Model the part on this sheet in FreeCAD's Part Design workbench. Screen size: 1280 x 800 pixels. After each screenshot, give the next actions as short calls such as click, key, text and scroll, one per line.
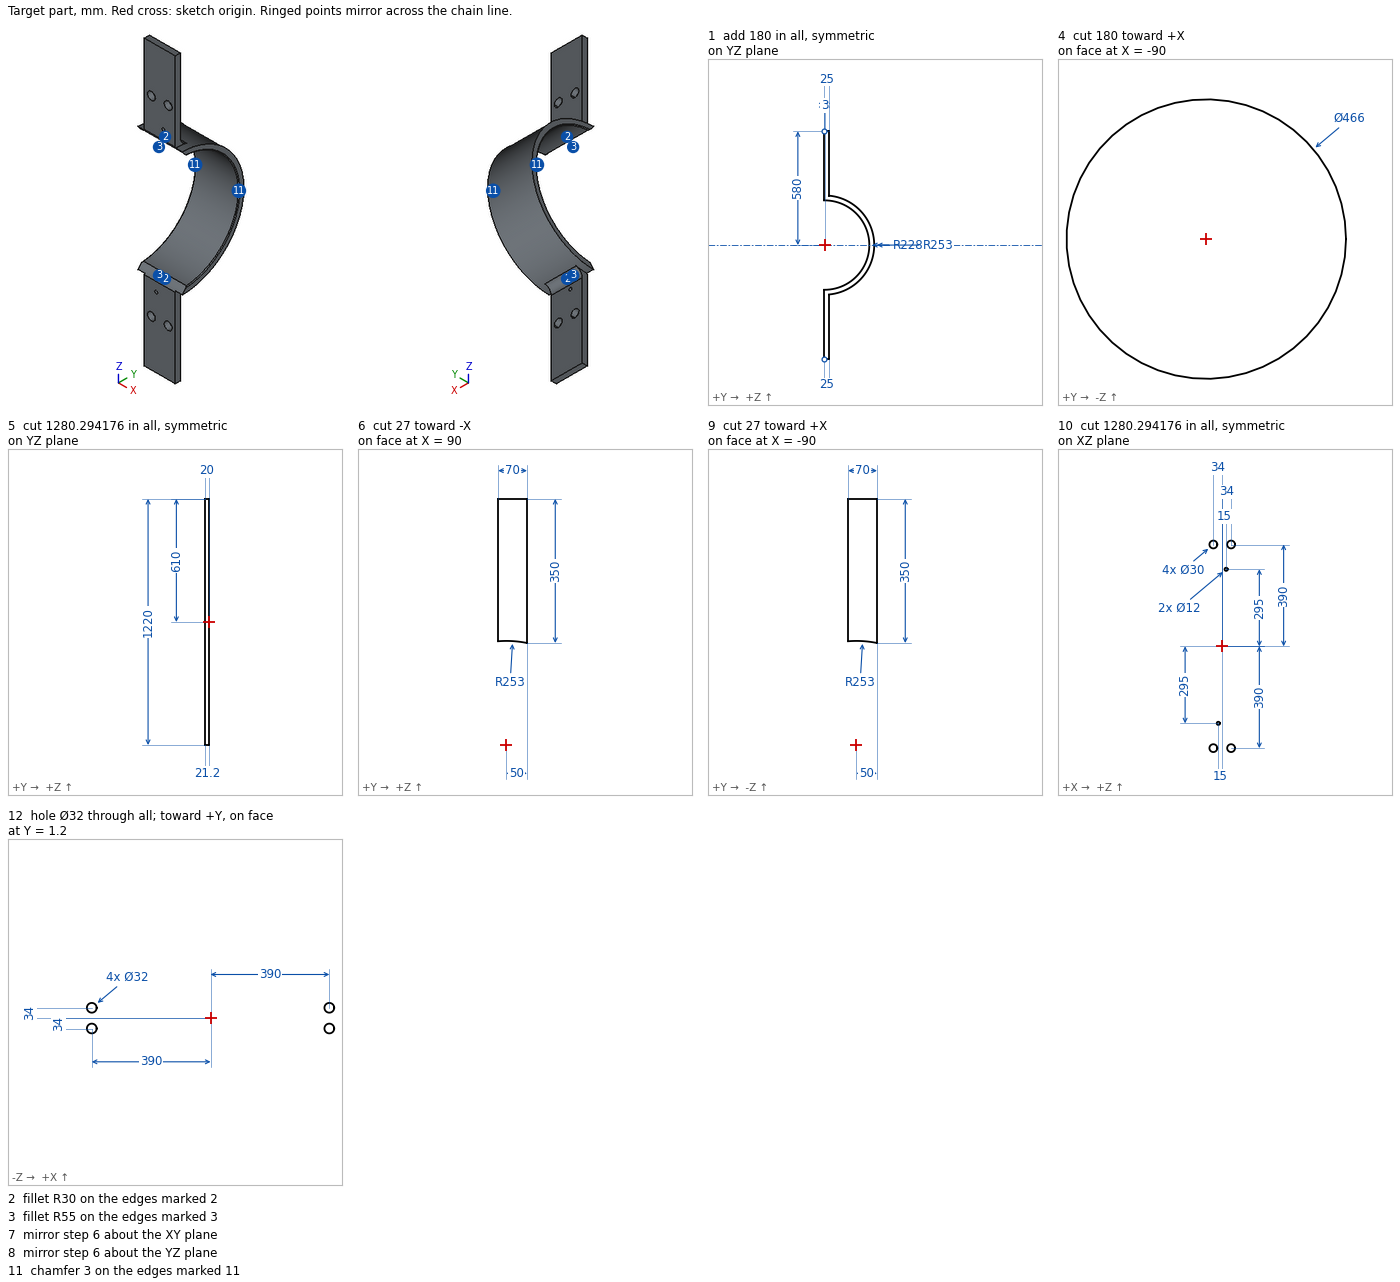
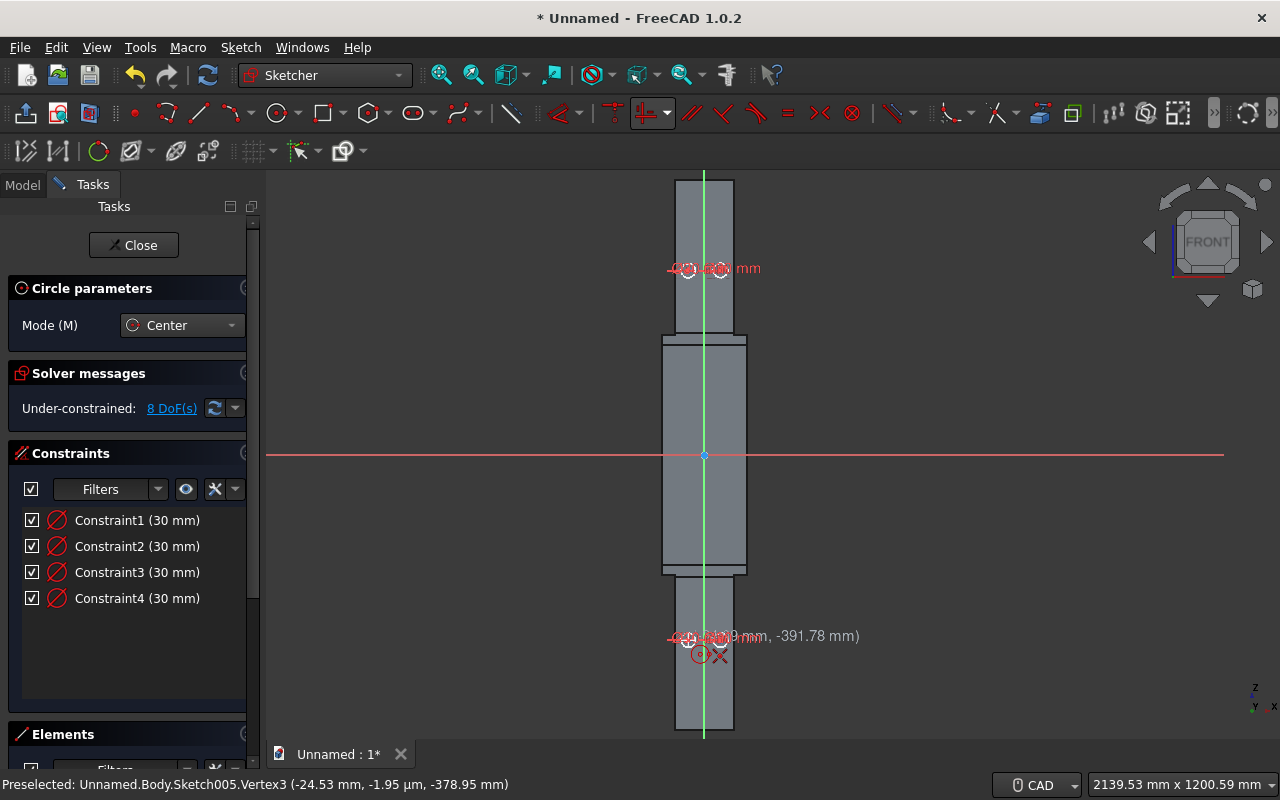
scroll(712, 315, up, 11)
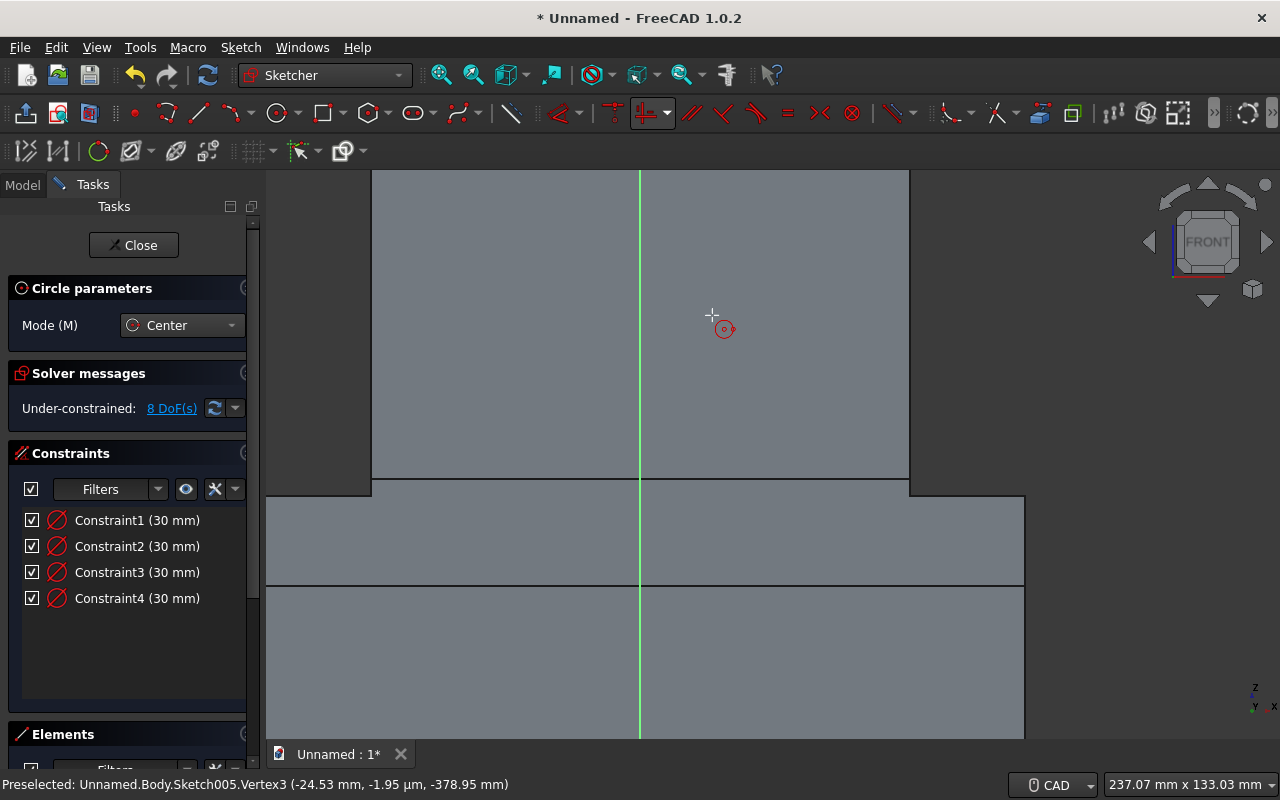
scroll(712, 314, down, 11)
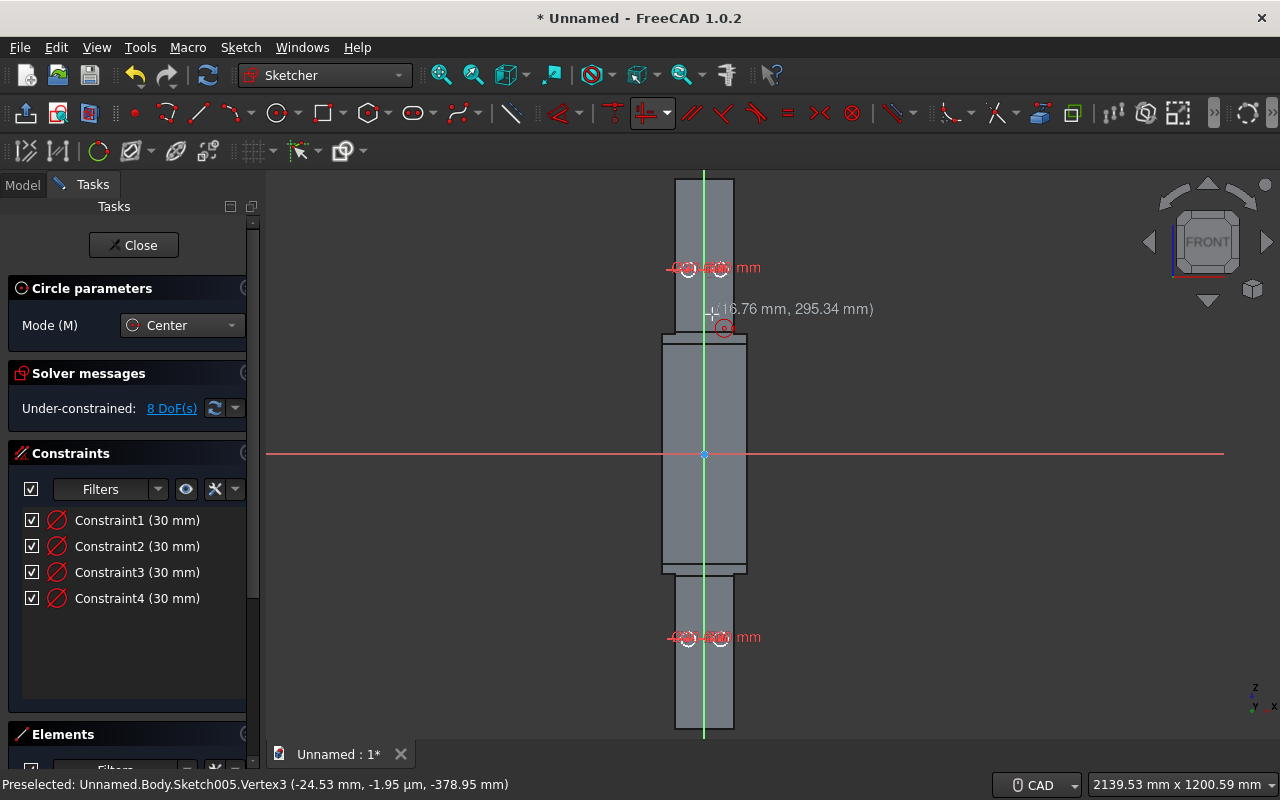
scroll(712, 314, up, 5)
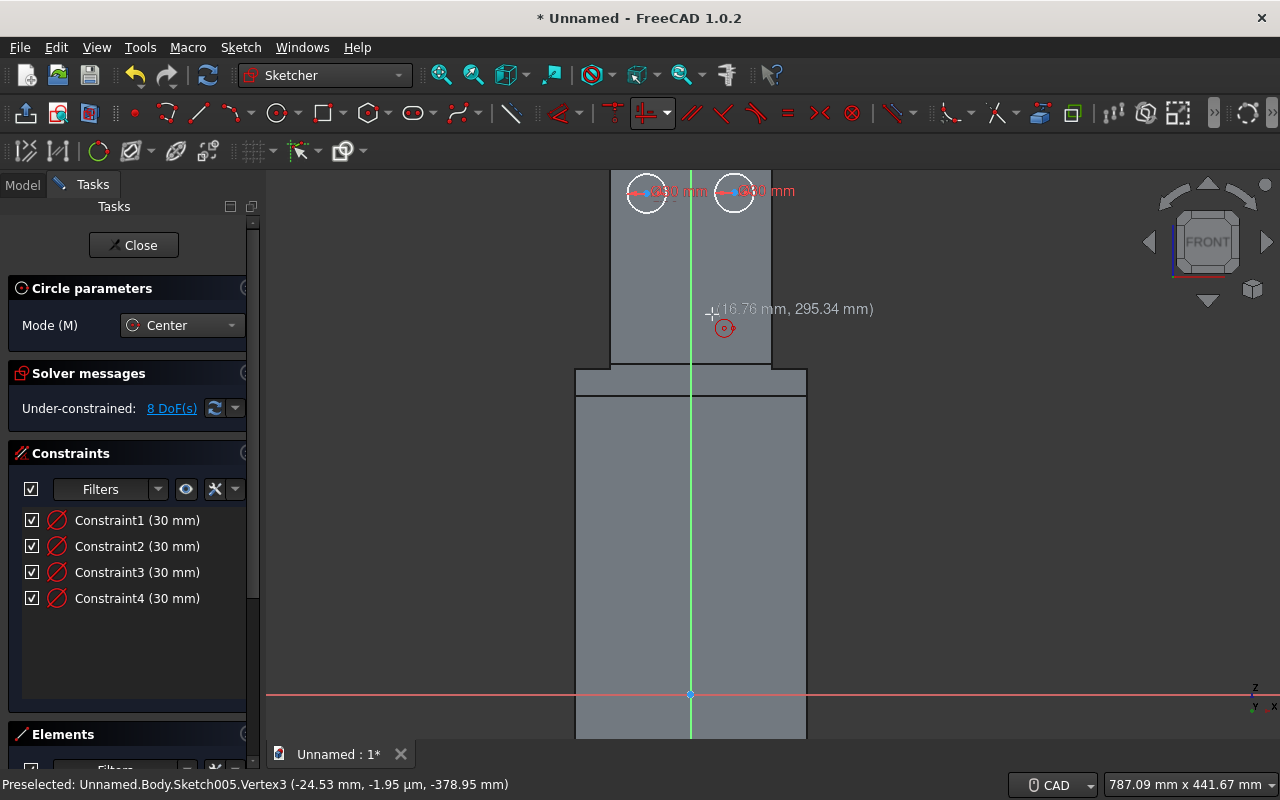
click(710, 315)
move(716, 309)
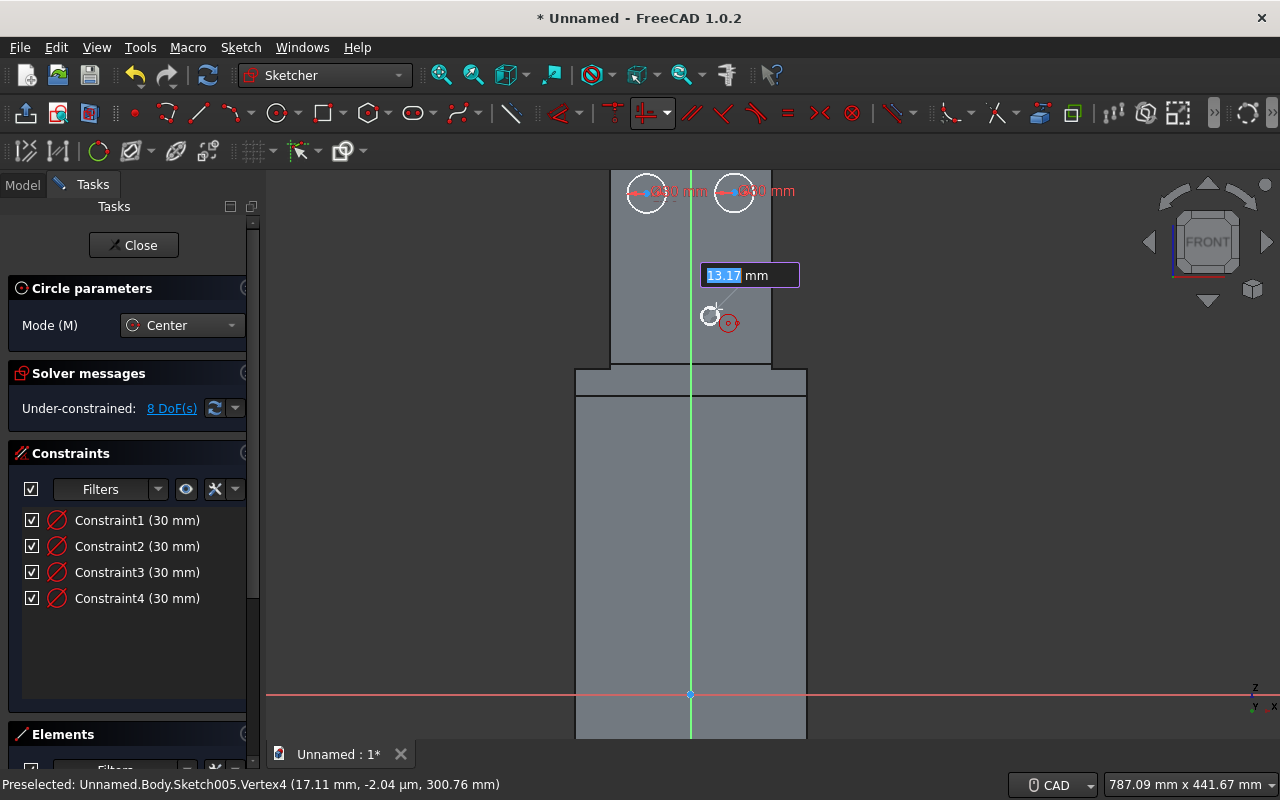
text(12)
key(Return)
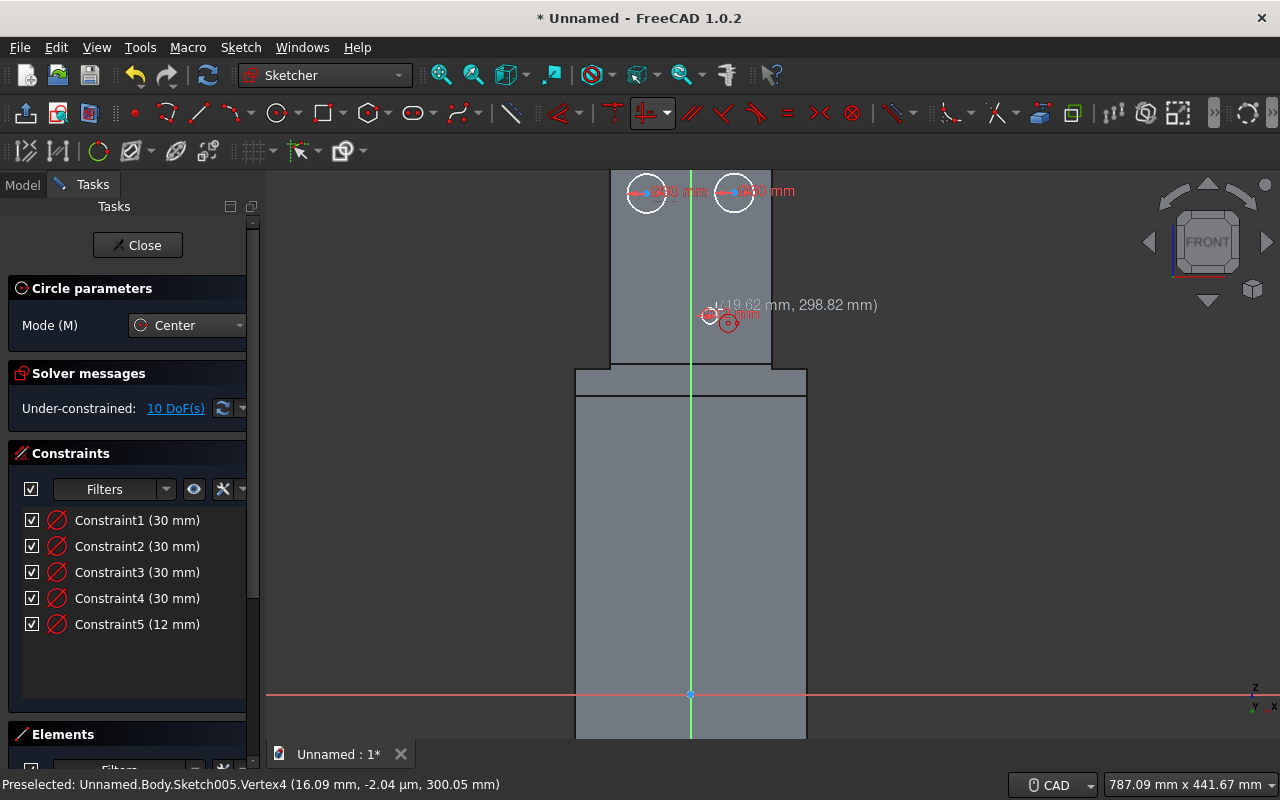
scroll(713, 315, down, 5)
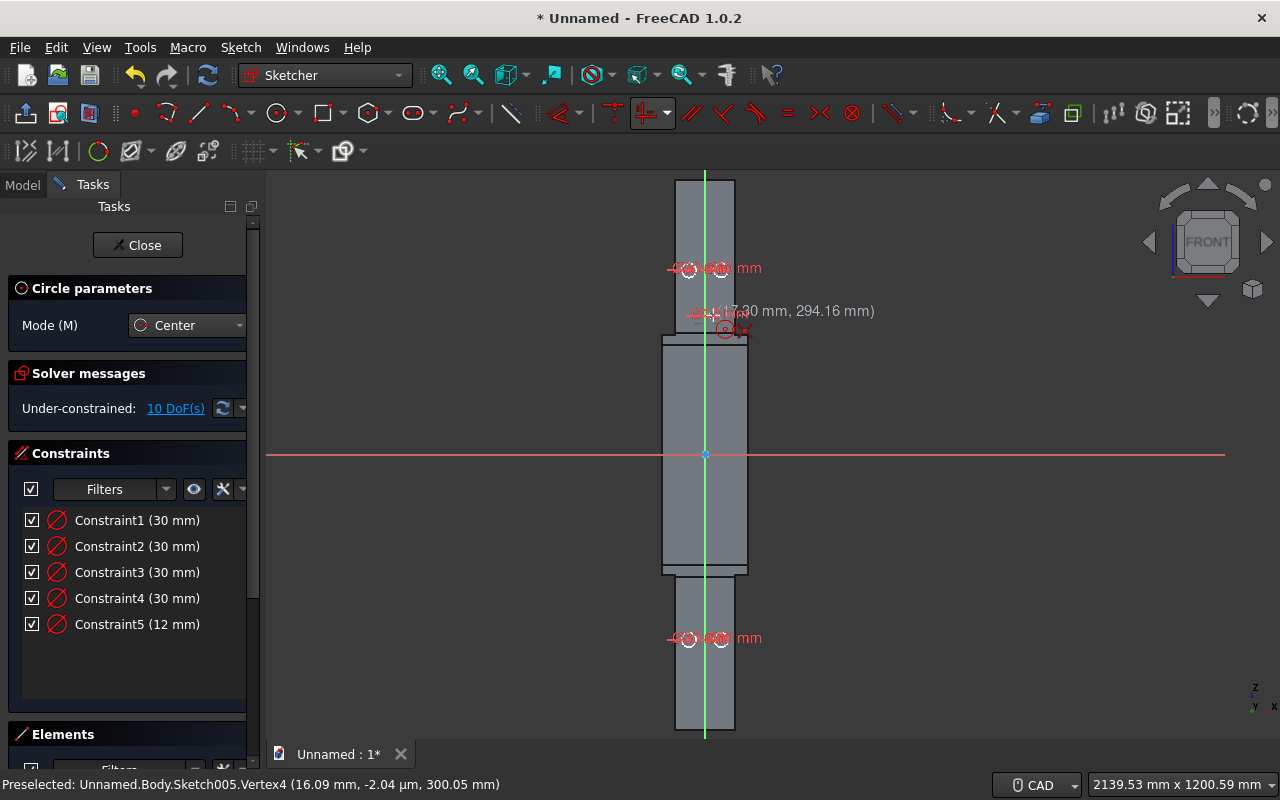
scroll(698, 595, up, 11)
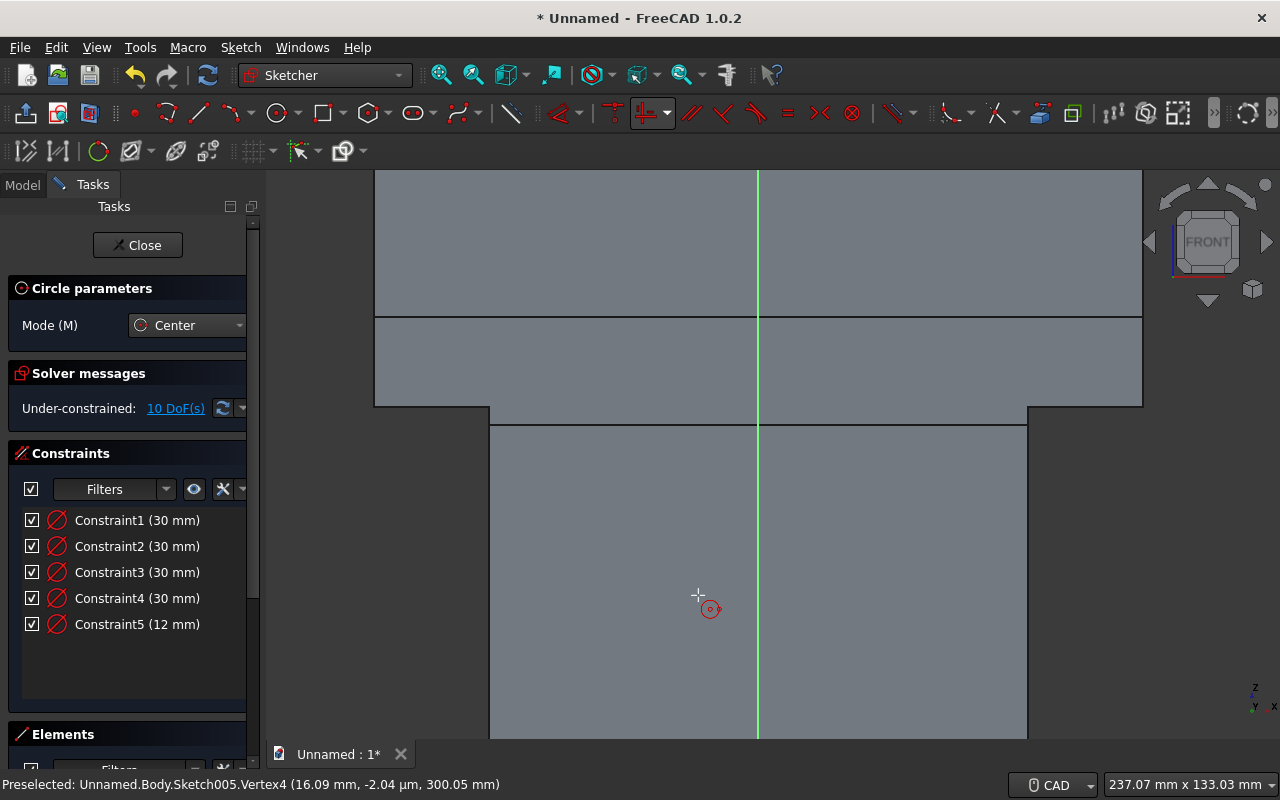
scroll(698, 595, down, 11)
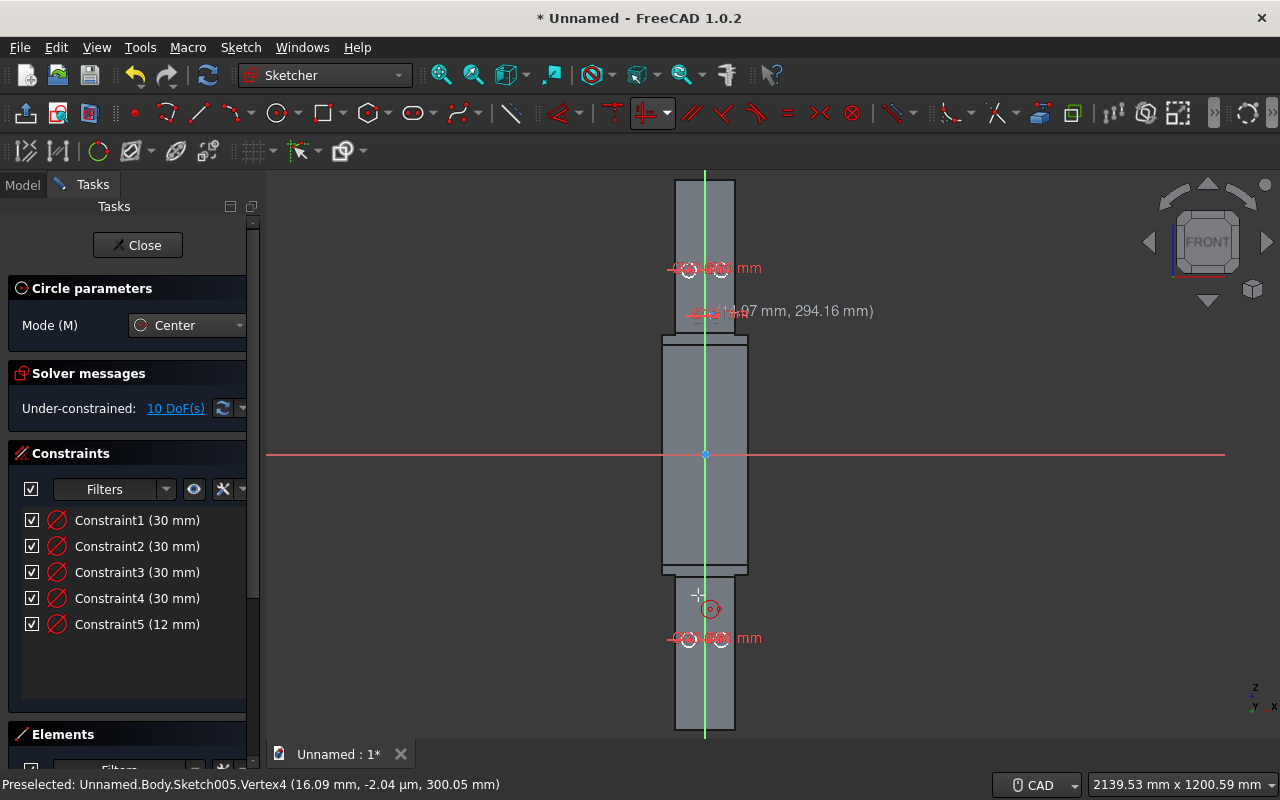
scroll(698, 595, up, 5)